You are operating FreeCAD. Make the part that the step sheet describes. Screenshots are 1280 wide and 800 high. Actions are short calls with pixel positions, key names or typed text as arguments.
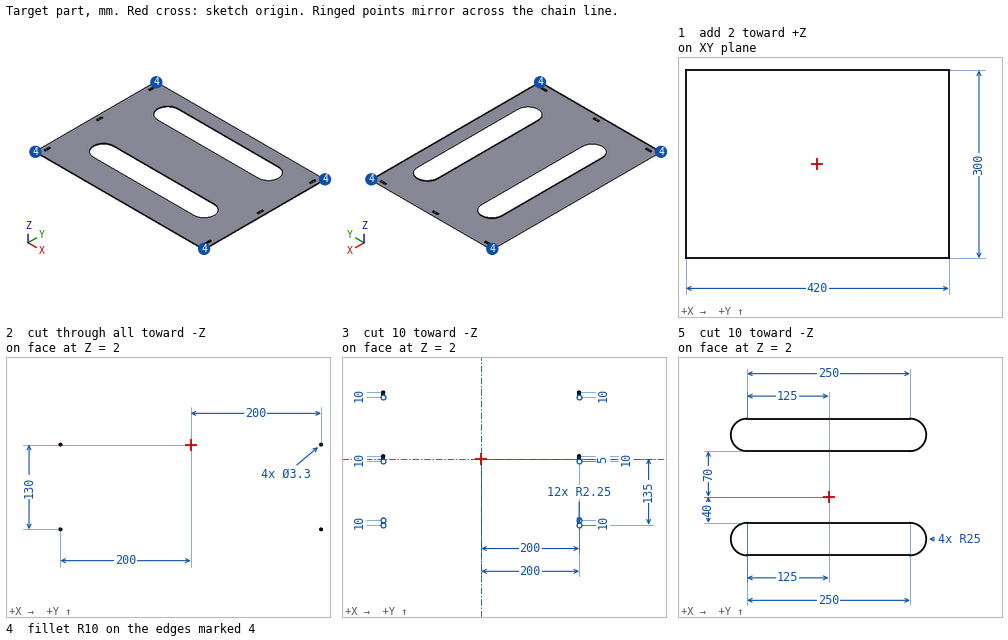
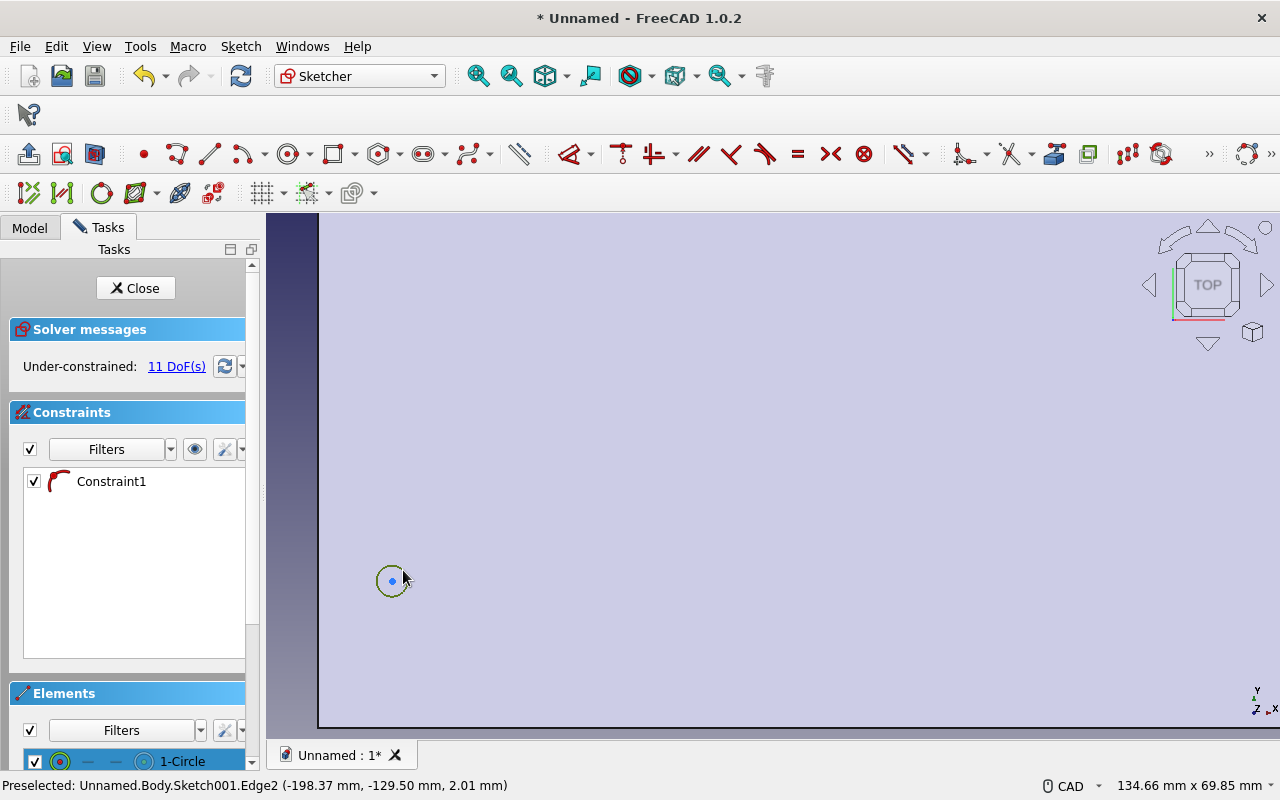
scroll(402, 574, down, 8)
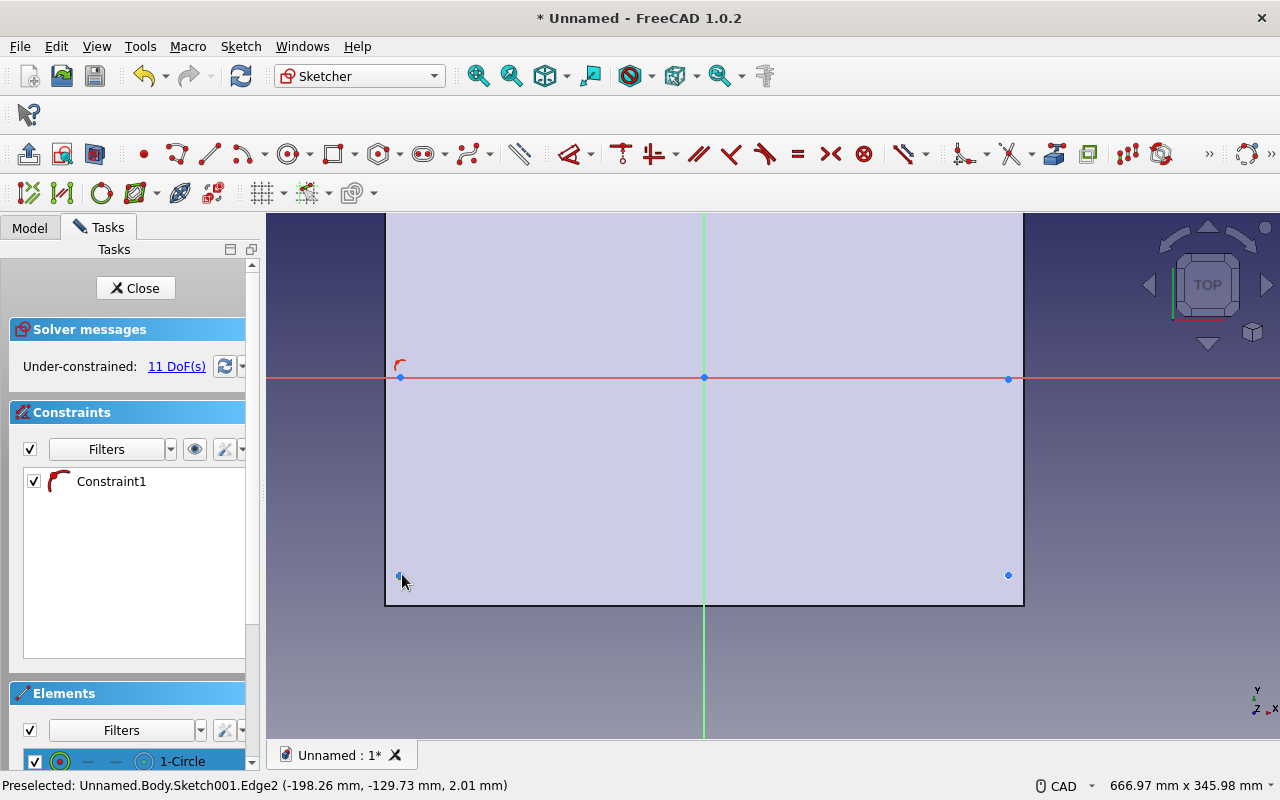
scroll(400, 375, up, 9)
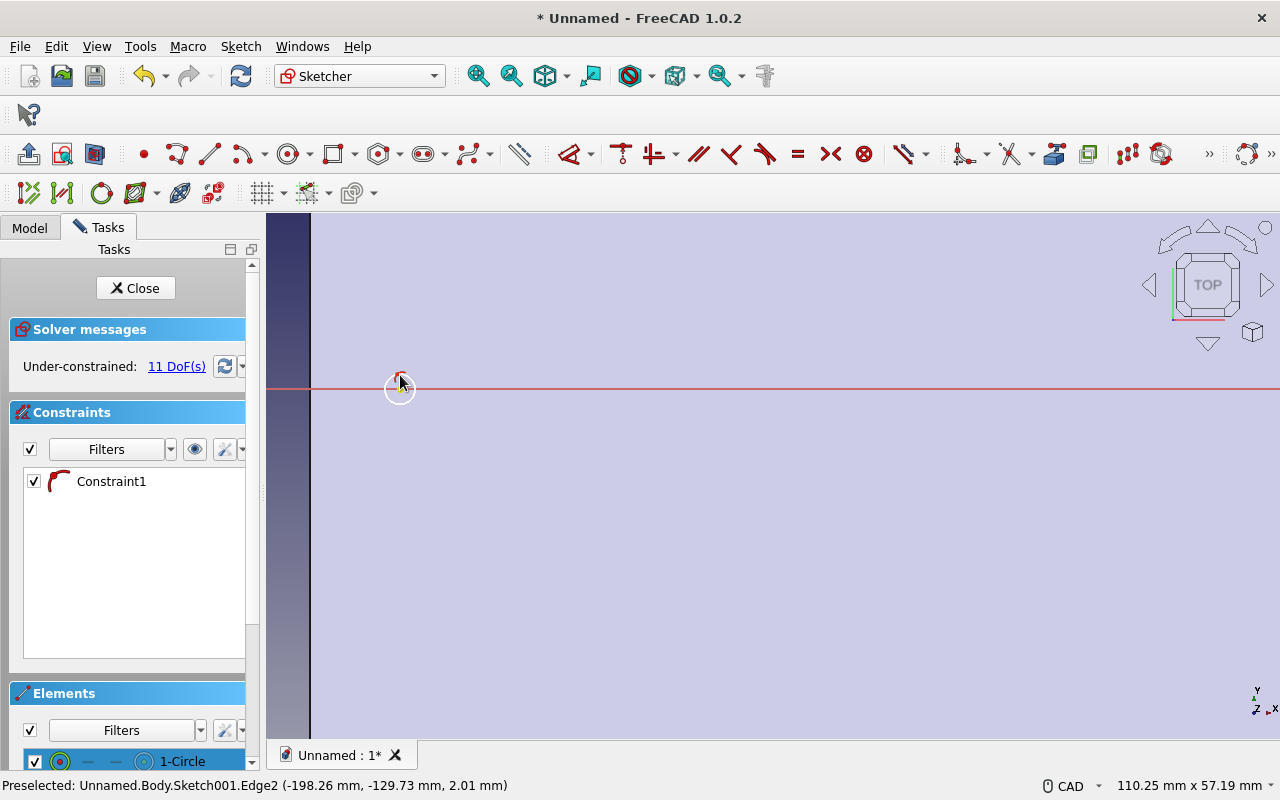
click(385, 389)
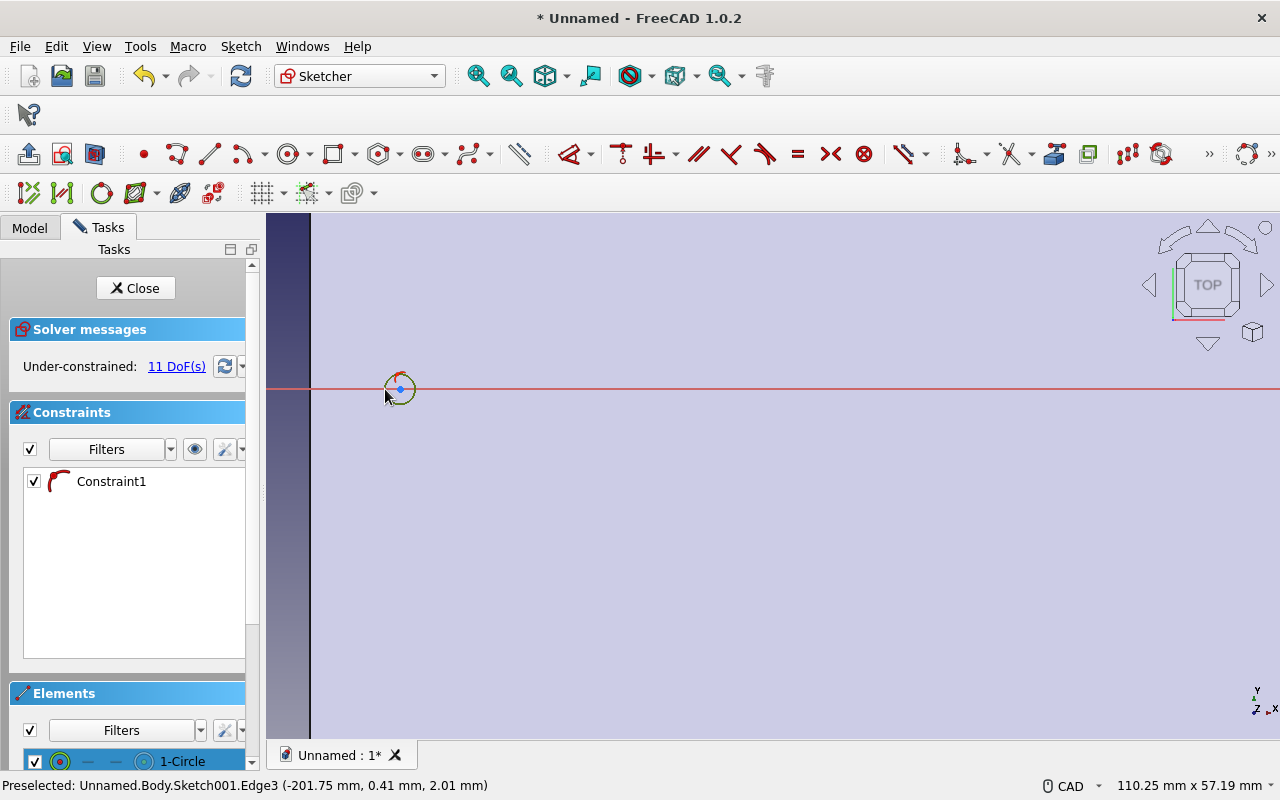
scroll(400, 375, down, 9)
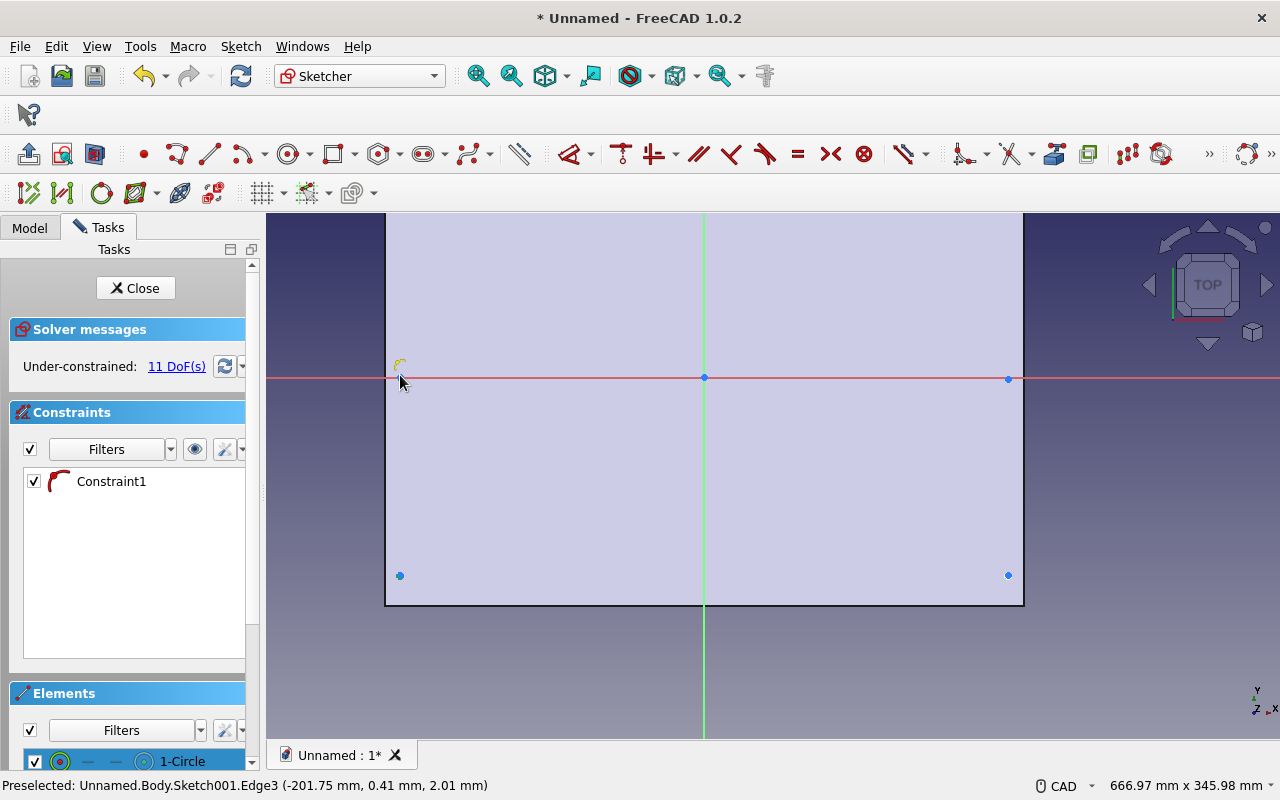
scroll(1010, 574, up, 8)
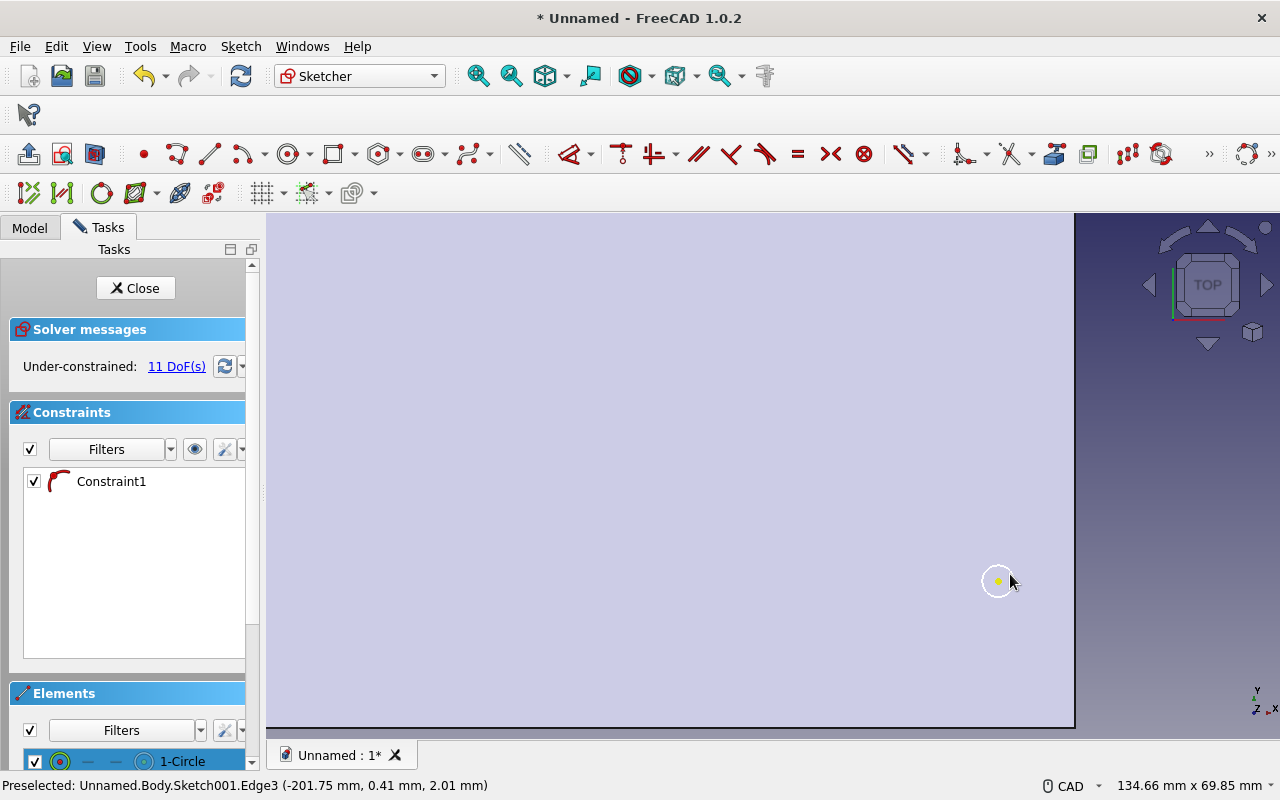
click(1009, 570)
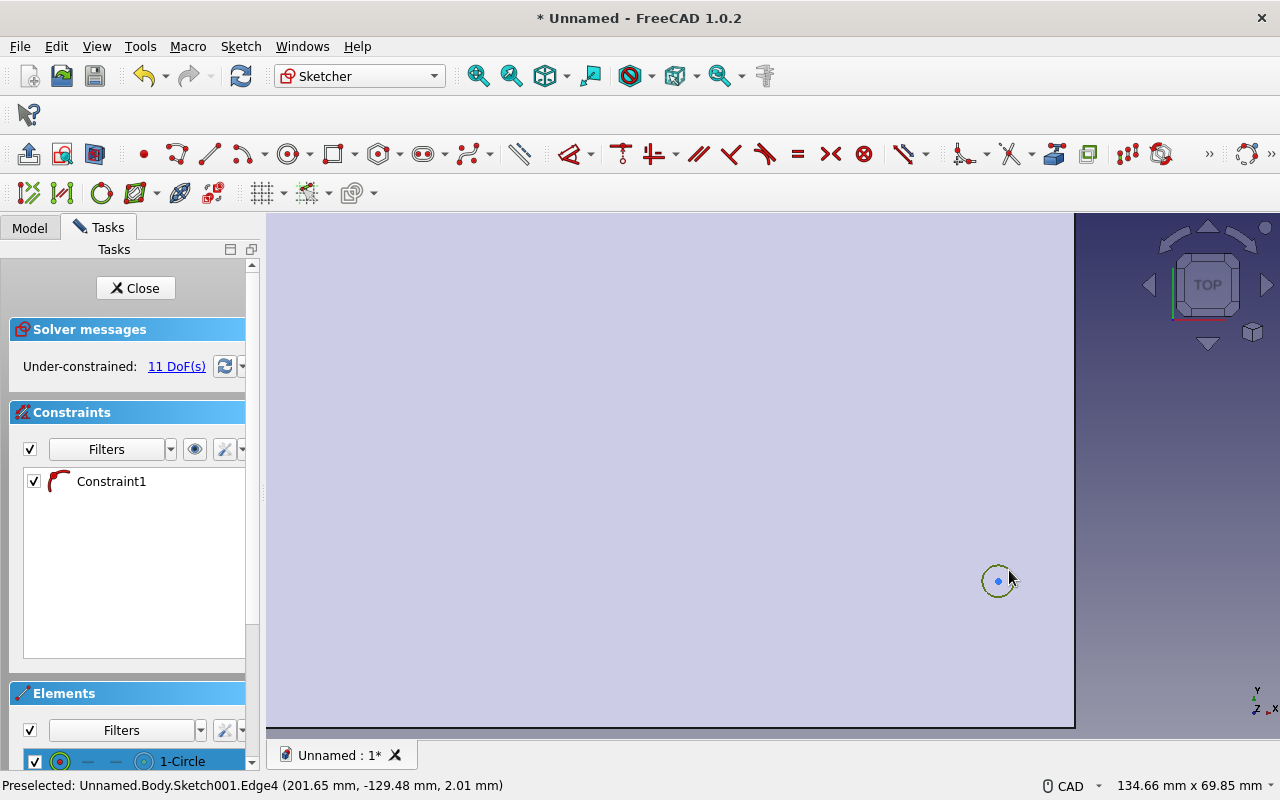
click(798, 154)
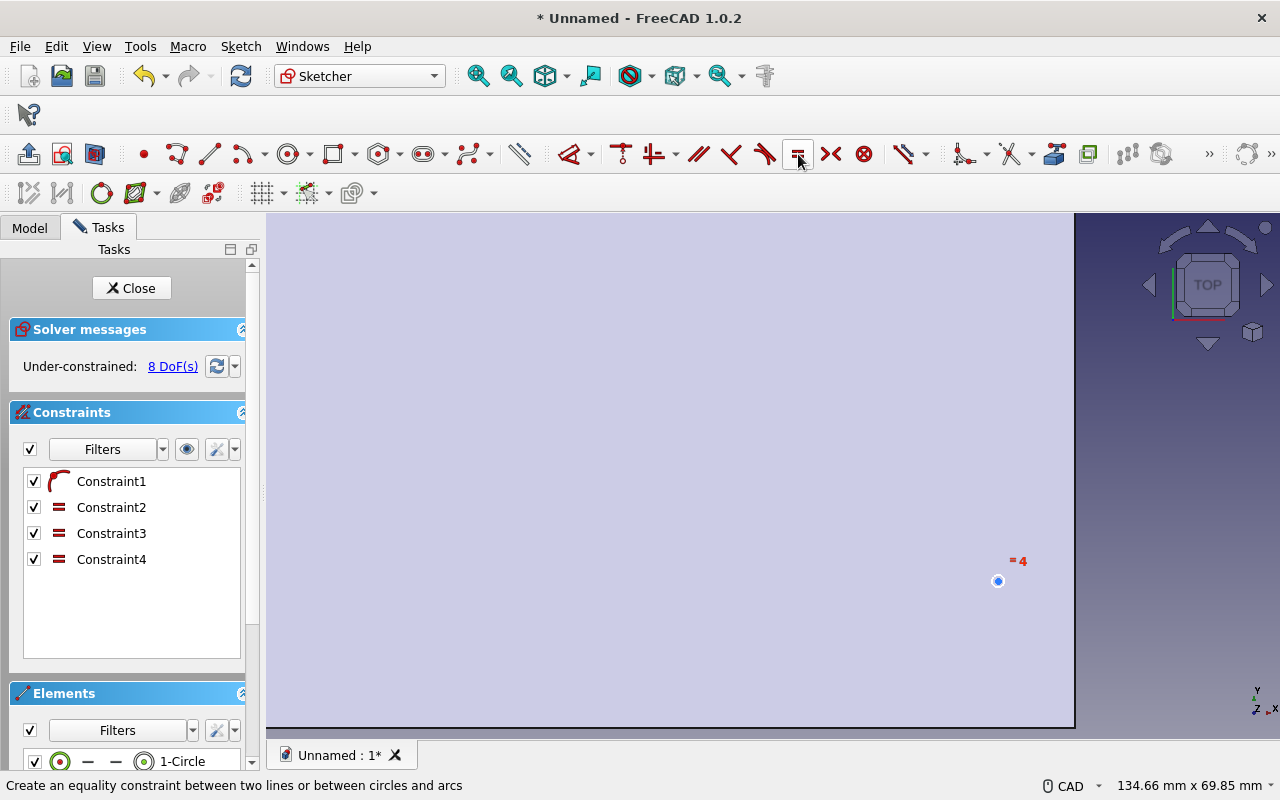
scroll(1011, 574, down, 8)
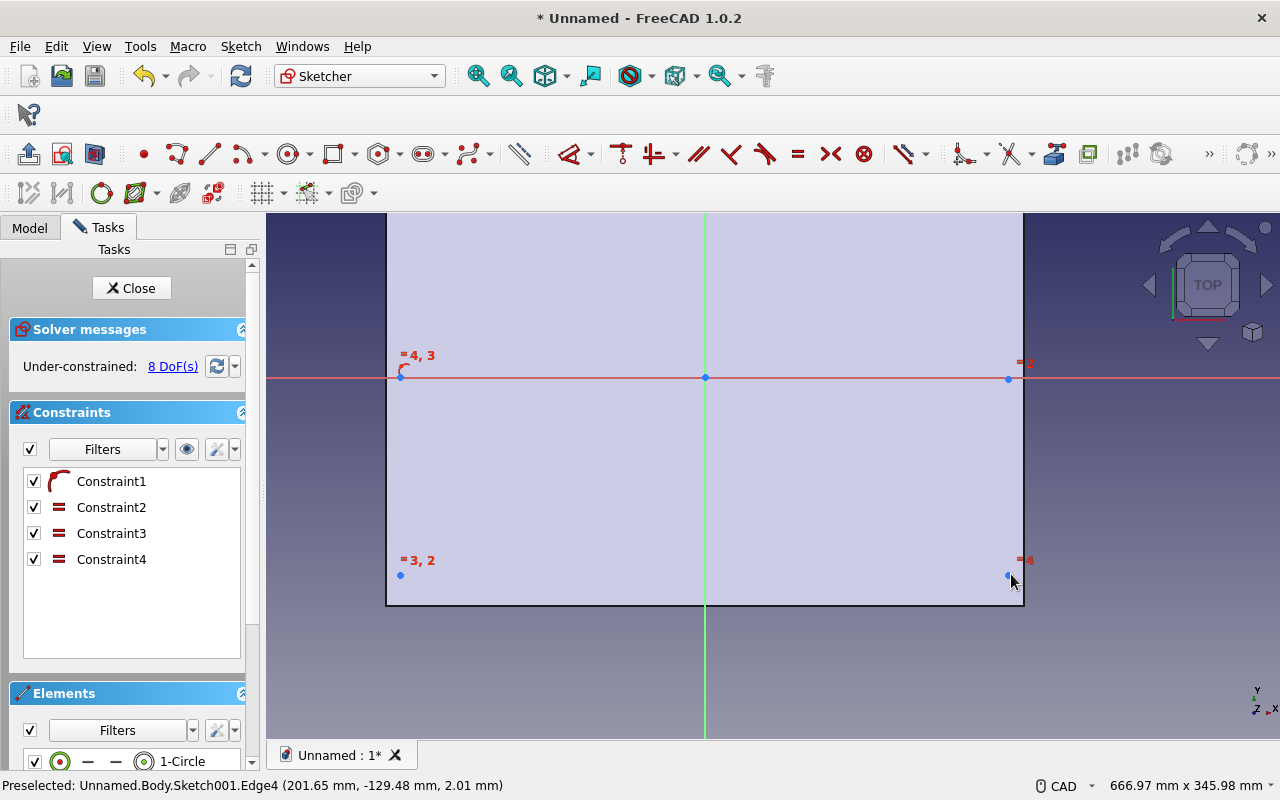
click(1009, 379)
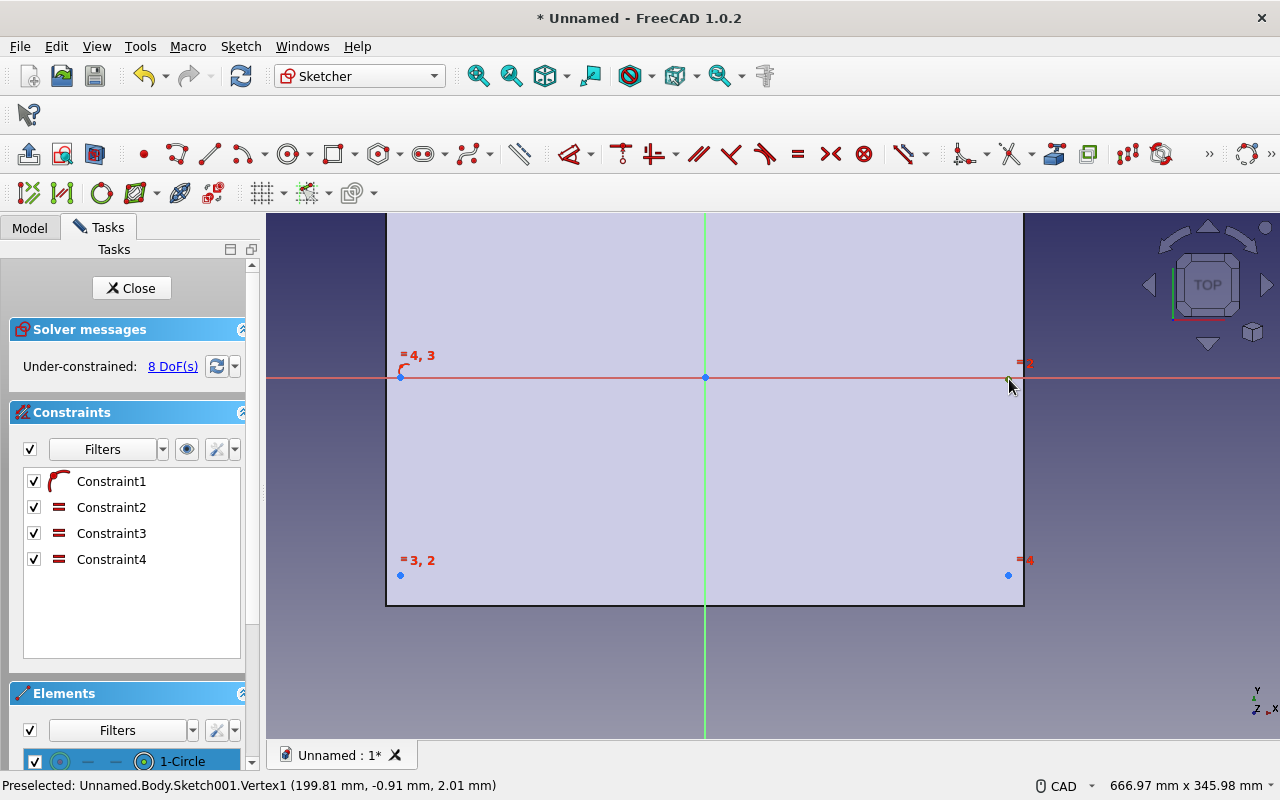
click(353, 378)